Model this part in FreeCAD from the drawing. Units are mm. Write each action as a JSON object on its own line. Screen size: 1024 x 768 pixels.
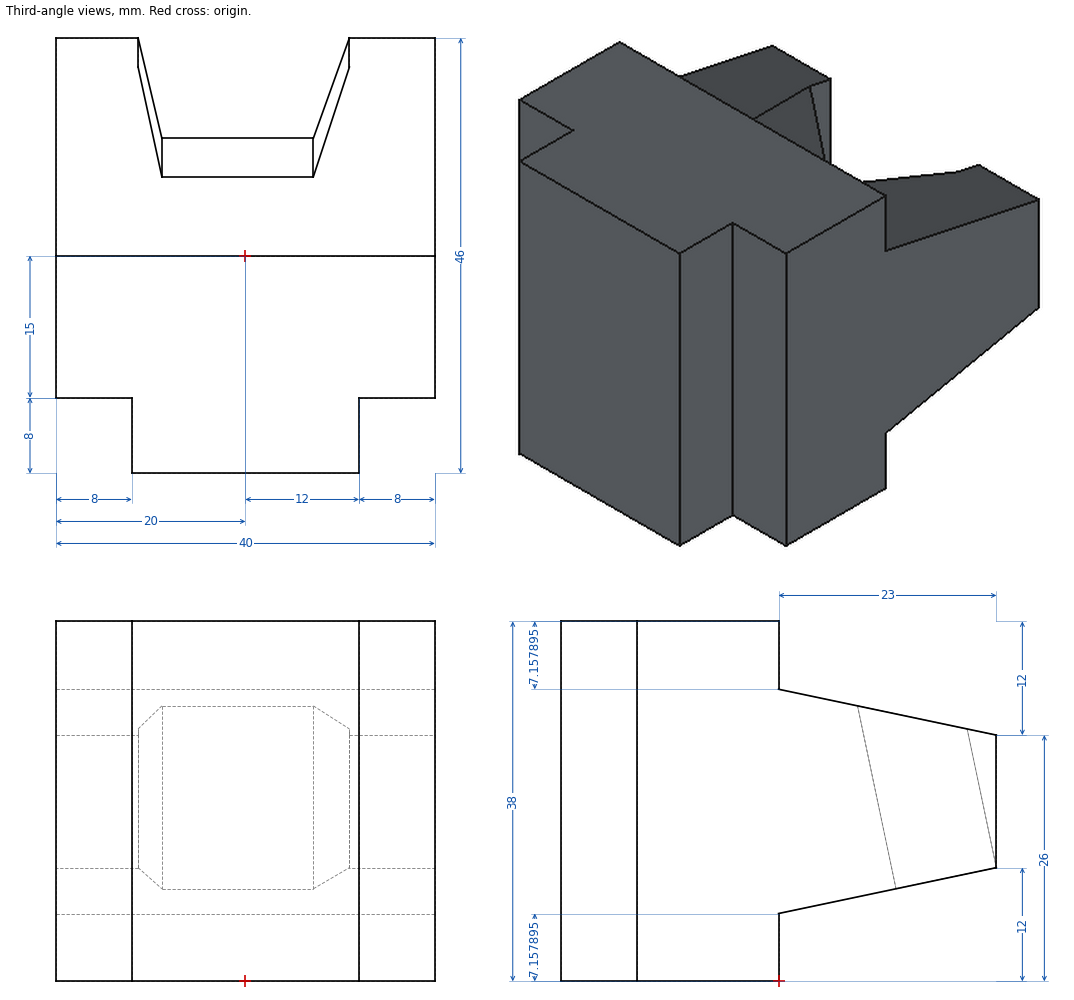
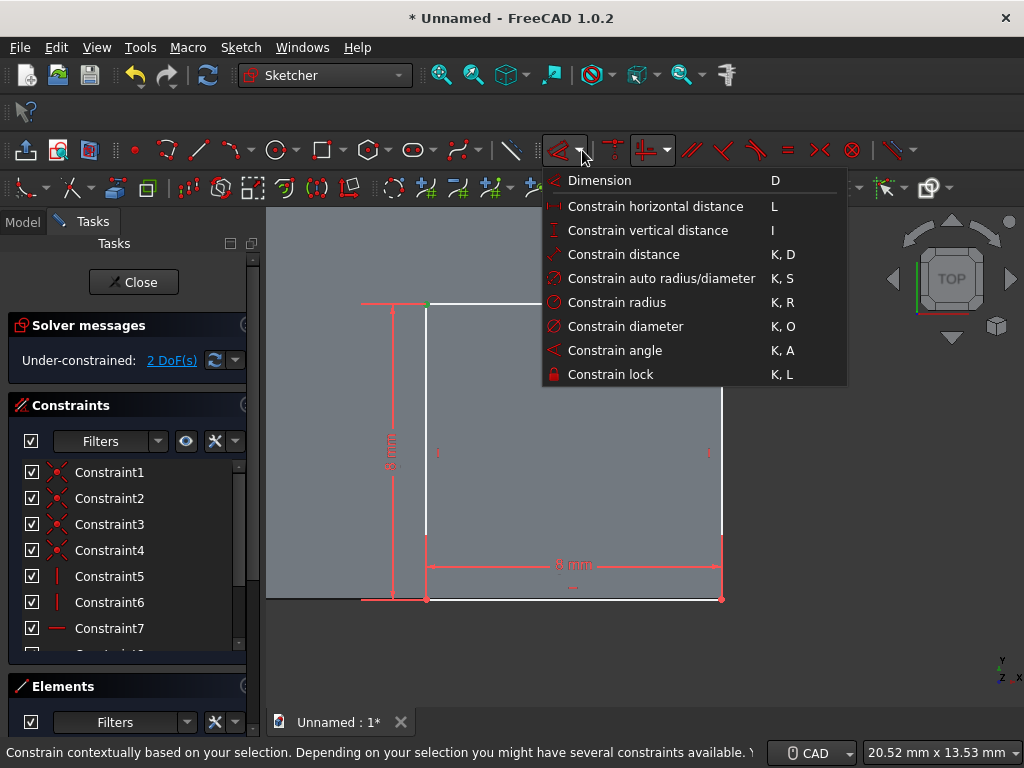
{"action": "left_click", "coordinate": [695, 206]}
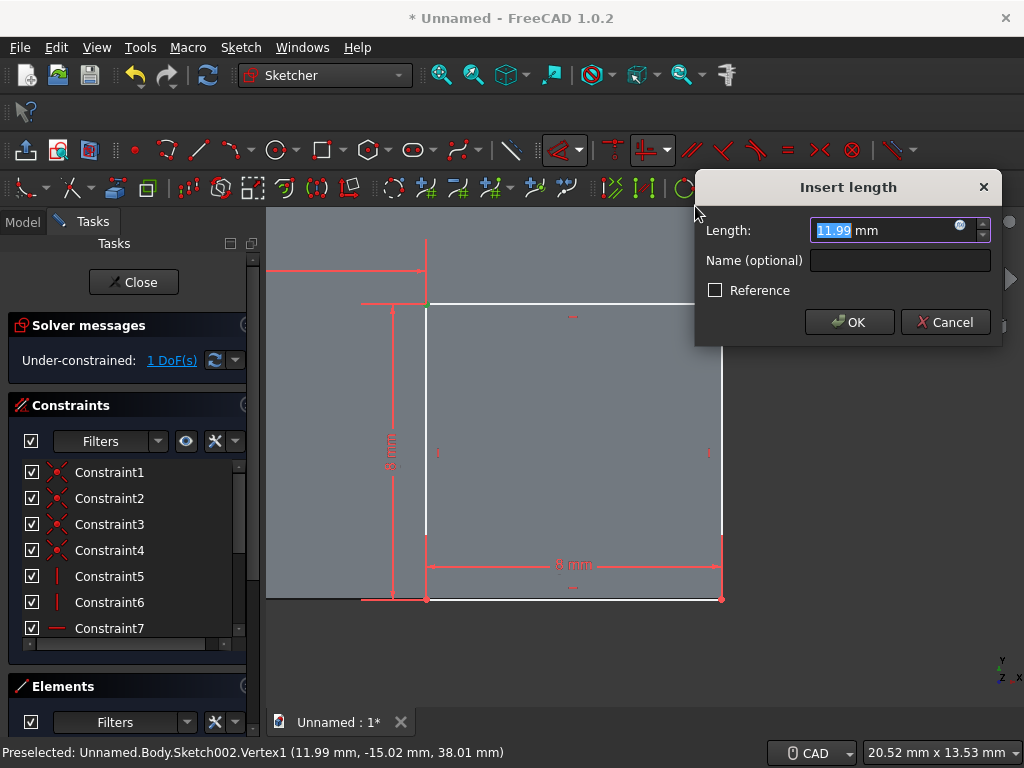
{"action": "type", "text": "12"}
{"action": "key", "text": "Return"}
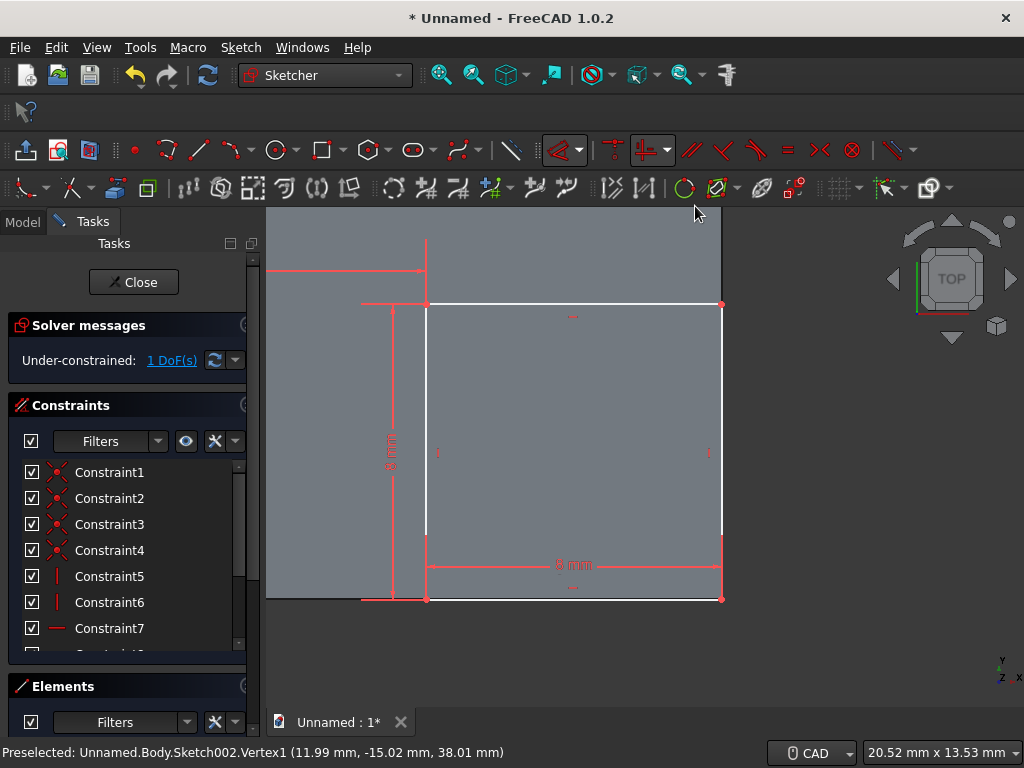
{"action": "left_click", "coordinate": [426, 304]}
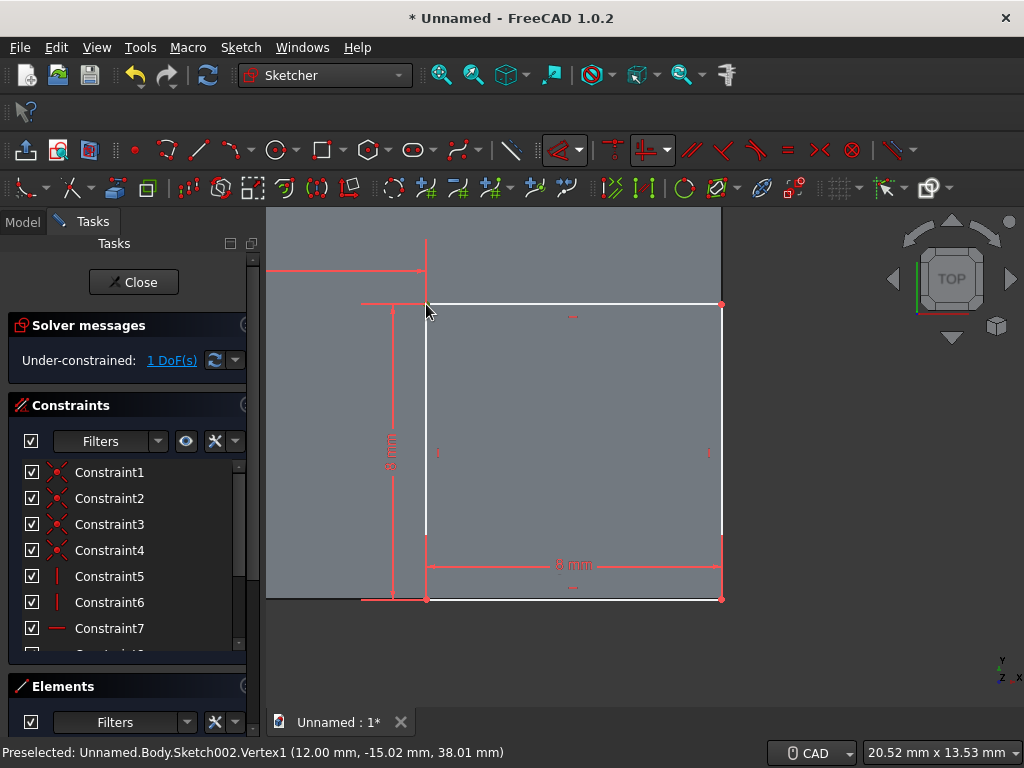
{"action": "key", "text": "i"}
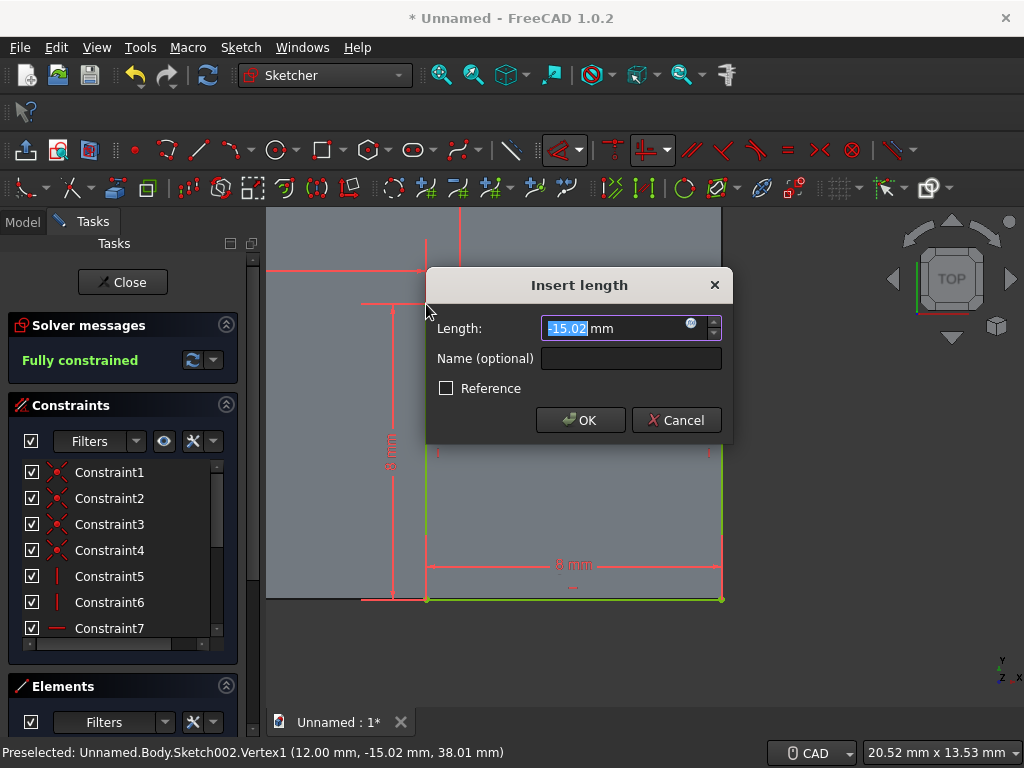
{"action": "type", "text": "-15"}
{"action": "key", "text": "Return"}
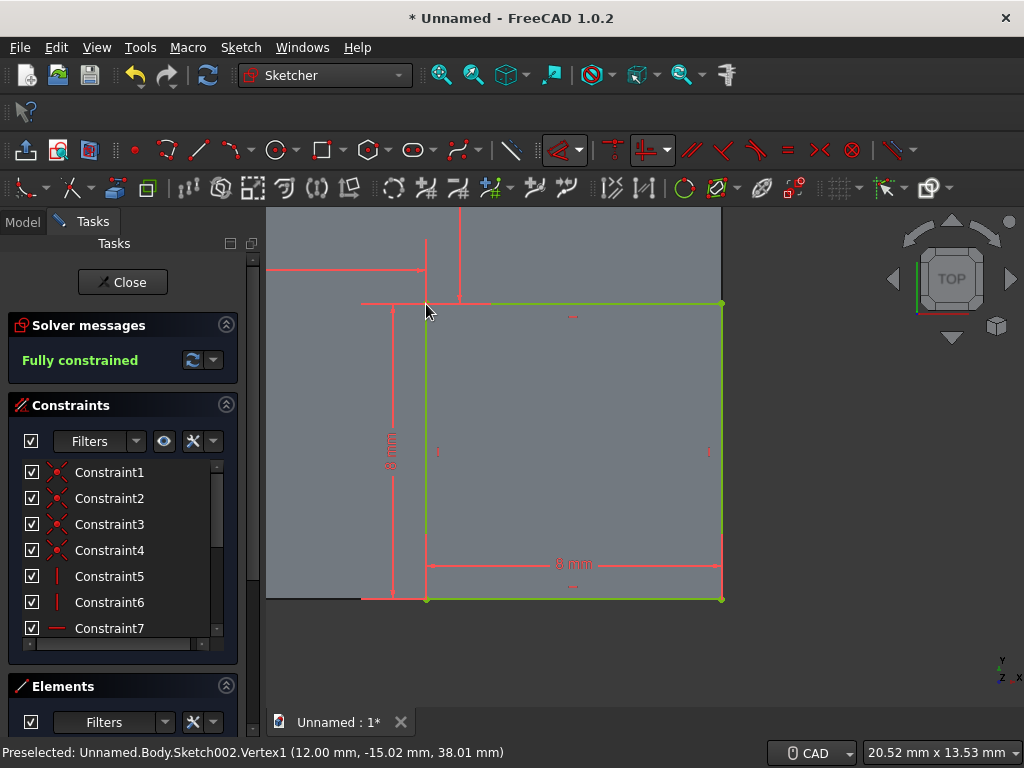
{"action": "left_click", "coordinate": [123, 282]}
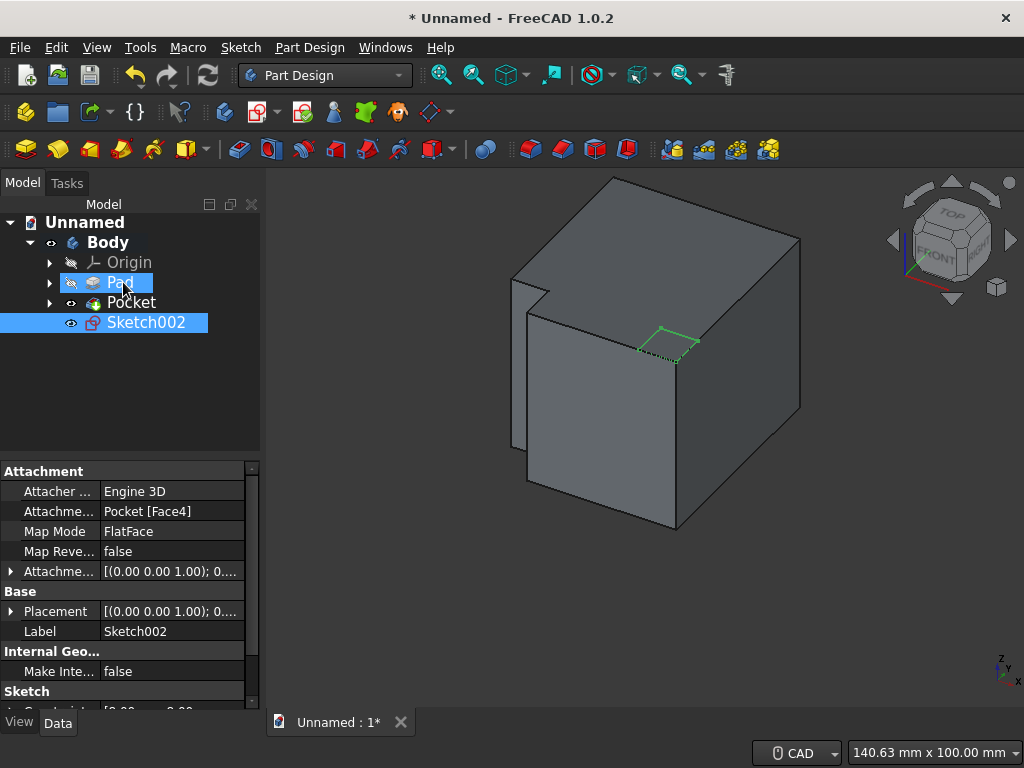
{"action": "left_click", "coordinate": [240, 150]}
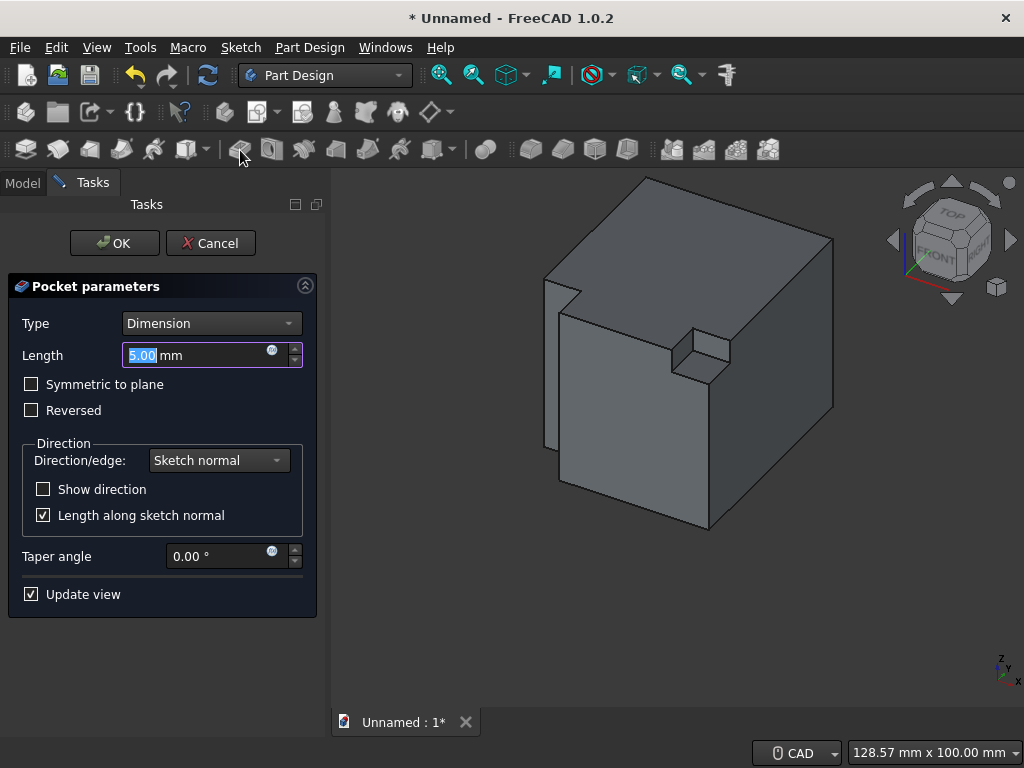
{"action": "left_click", "coordinate": [212, 324]}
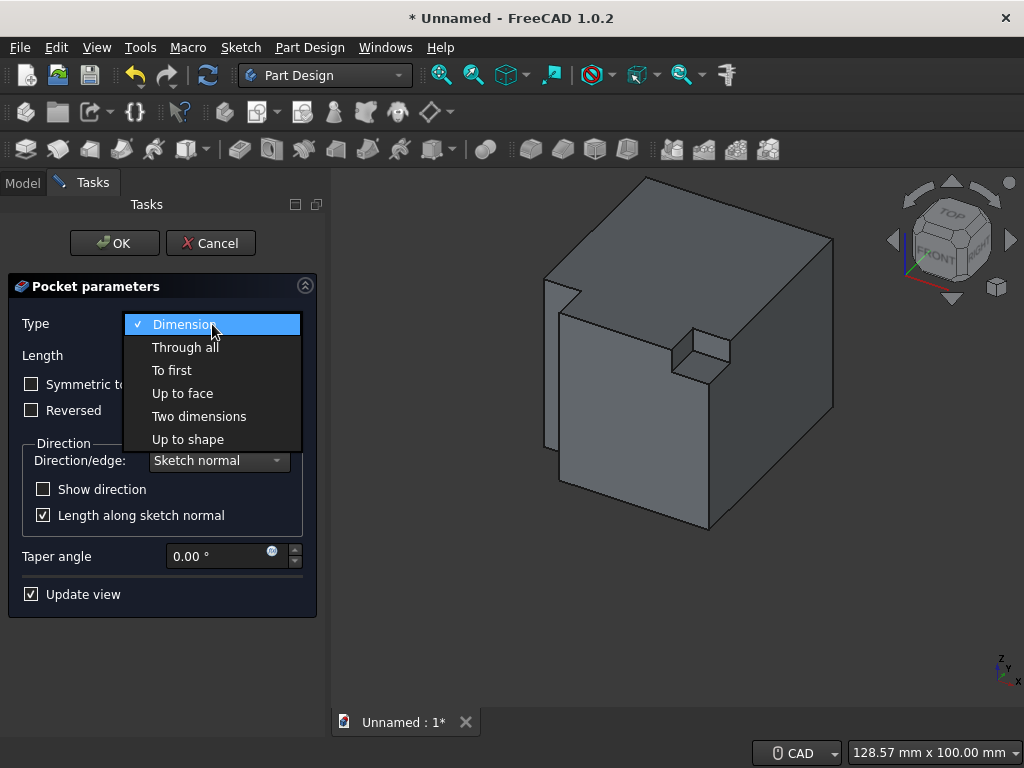
{"action": "left_click", "coordinate": [212, 348]}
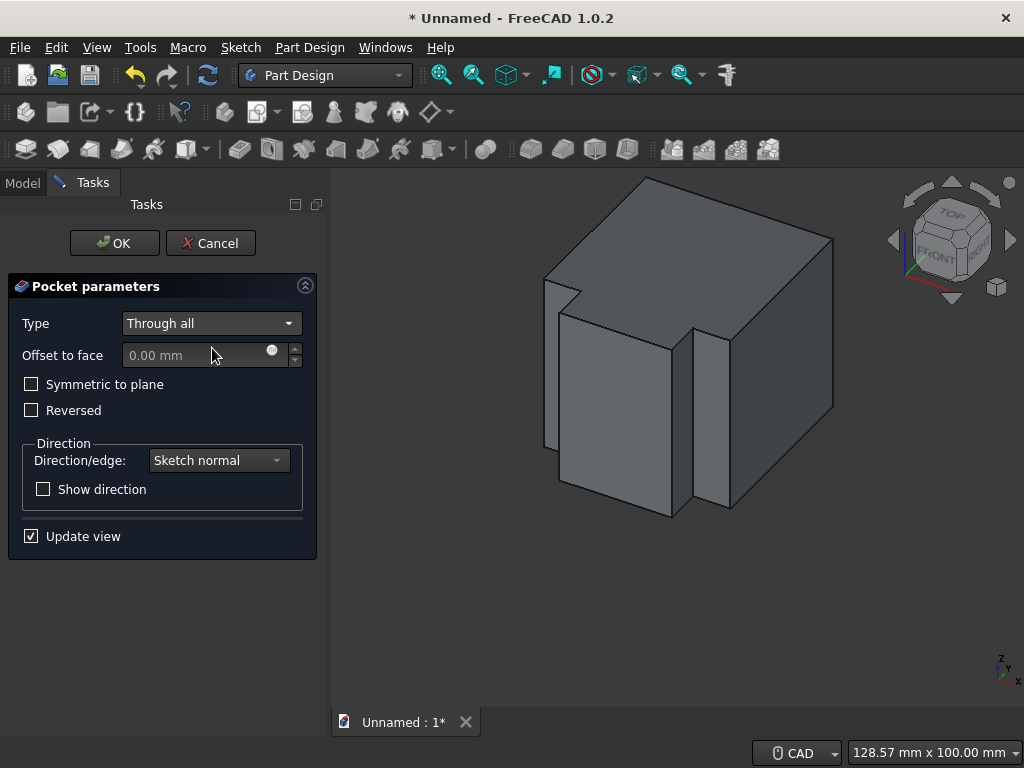
{"action": "left_click", "coordinate": [115, 243]}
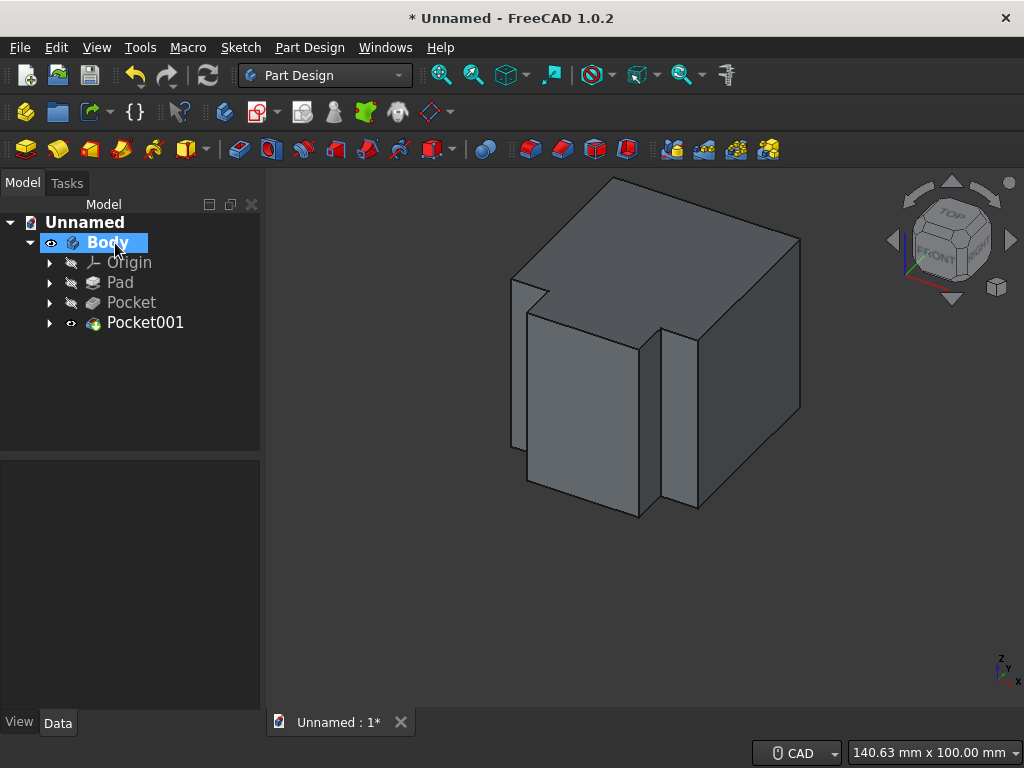
{"action": "left_click", "coordinate": [258, 112]}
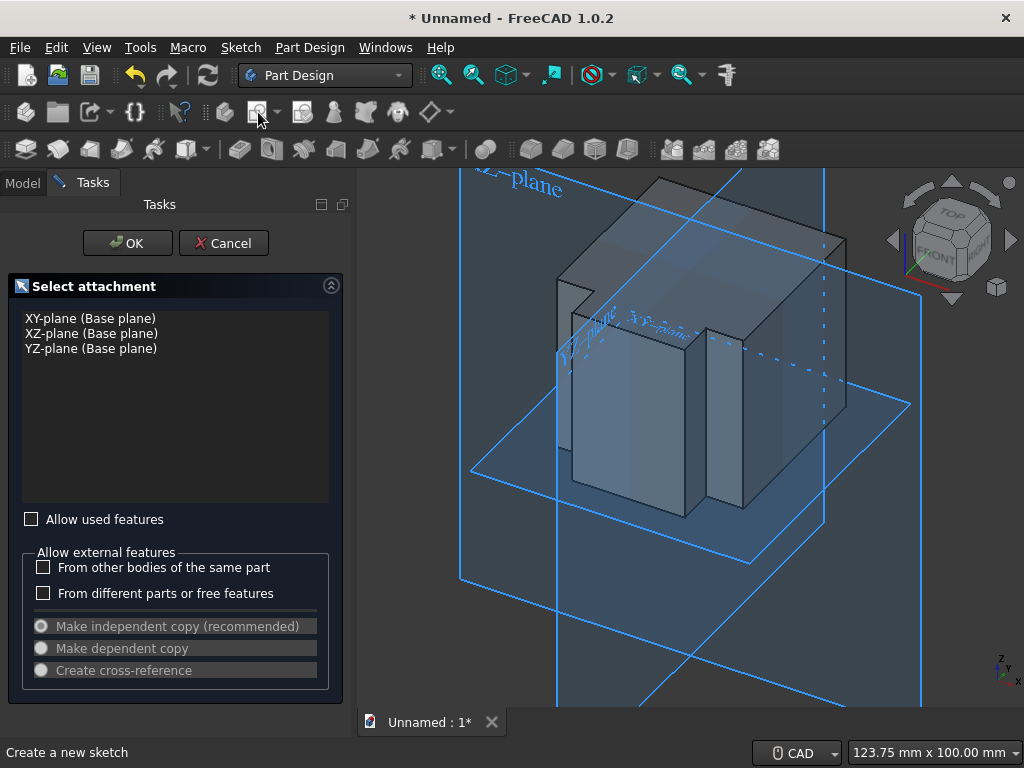
{"action": "left_click", "coordinate": [82, 348]}